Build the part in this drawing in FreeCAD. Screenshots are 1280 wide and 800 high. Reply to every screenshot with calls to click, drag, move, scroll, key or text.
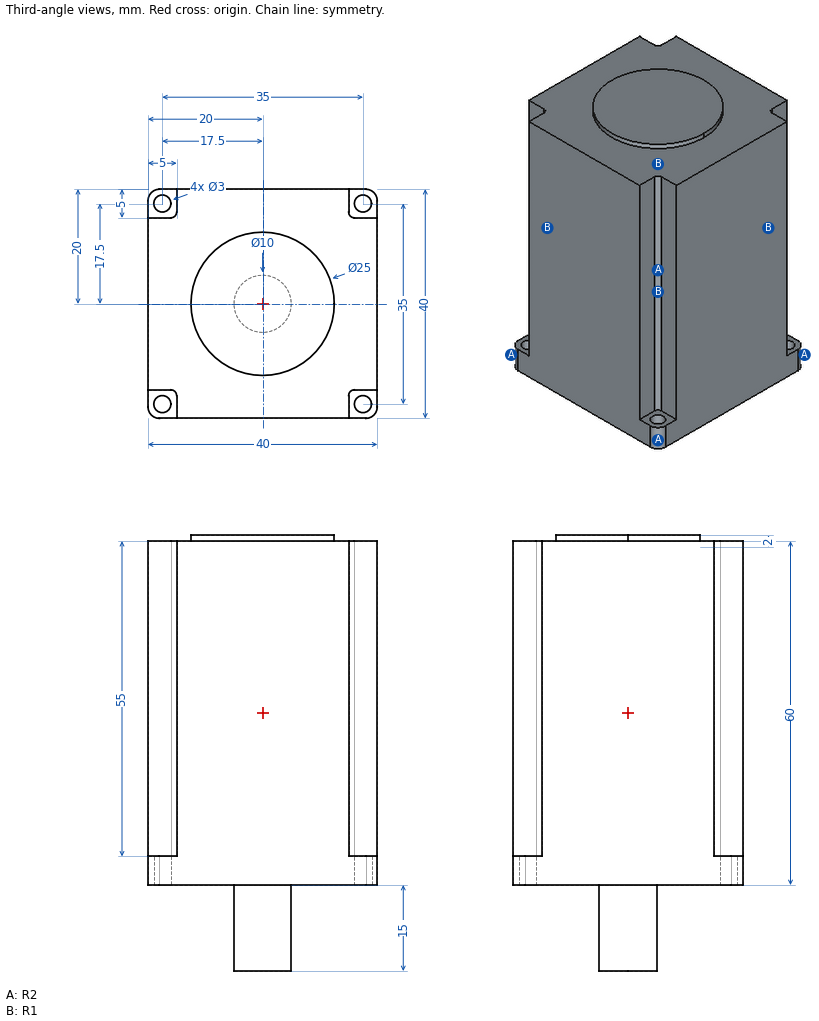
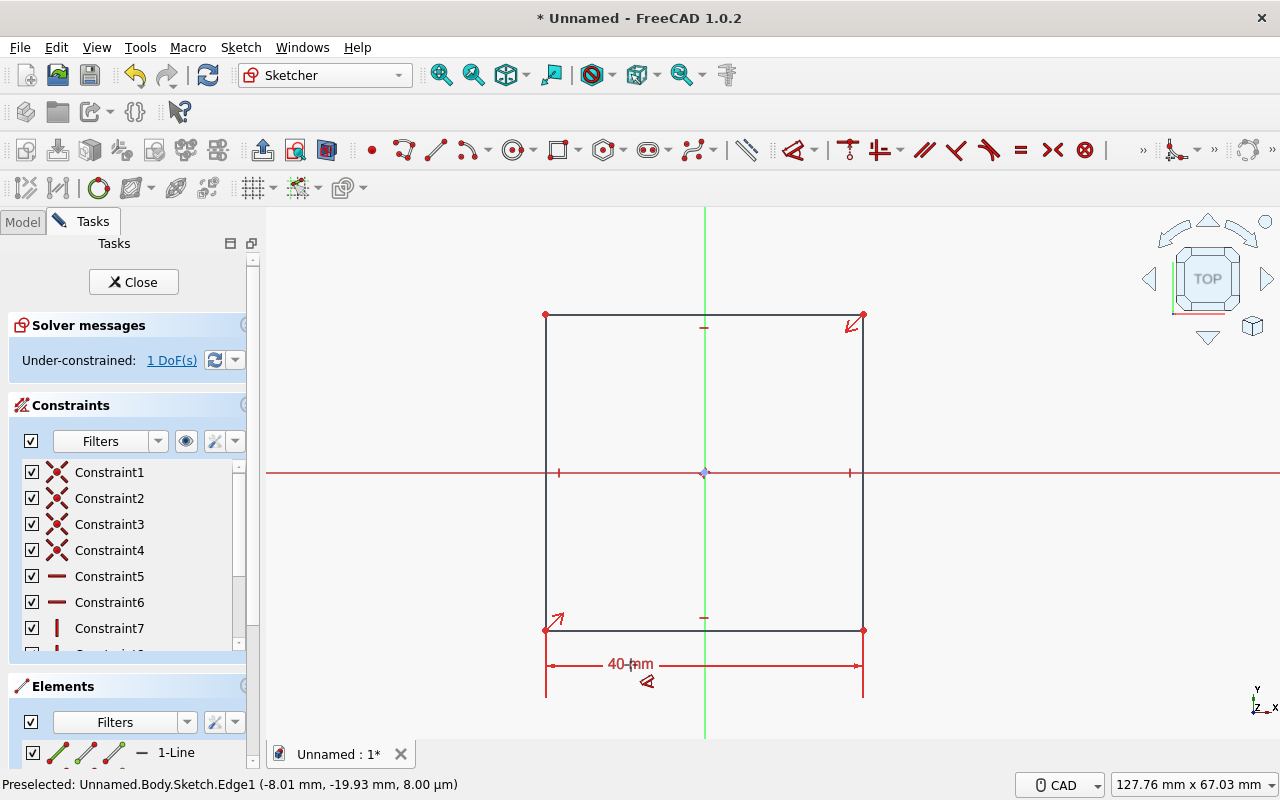
click(863, 536)
click(897, 400)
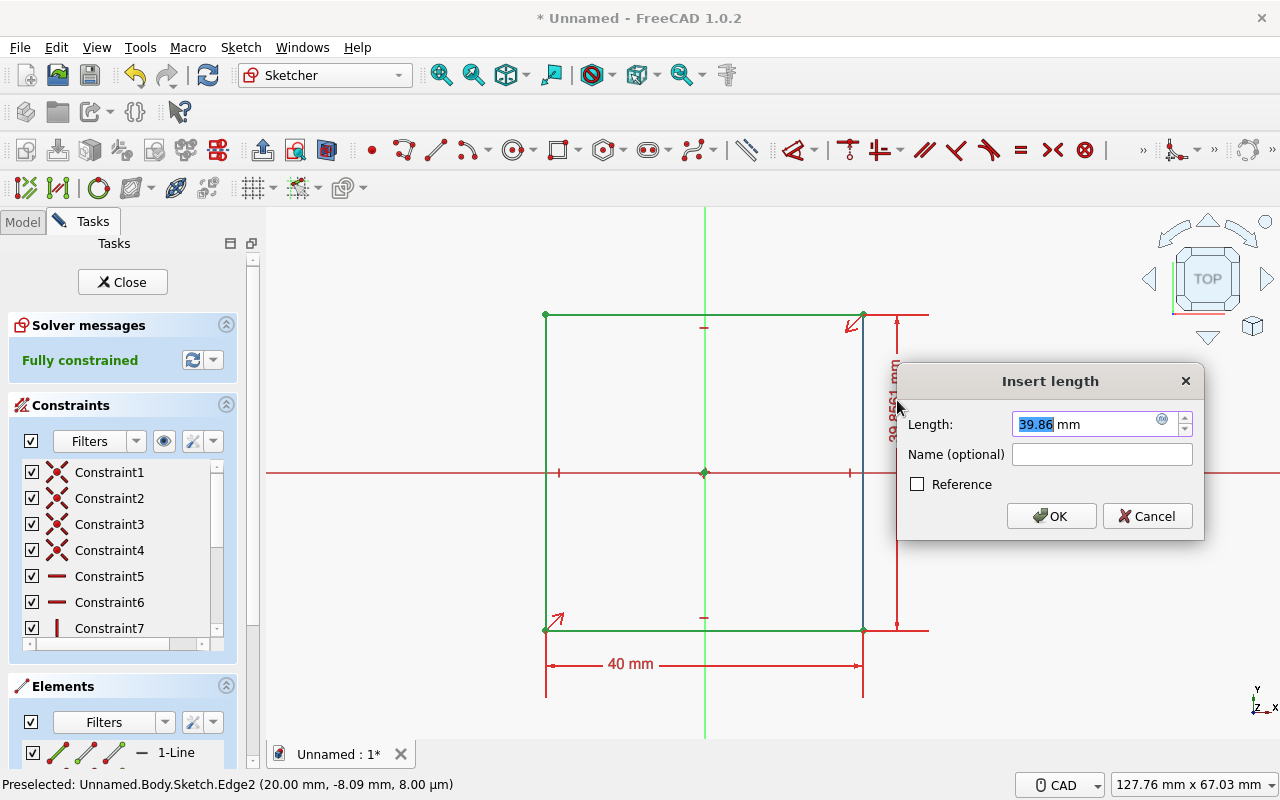
text(40)
key(Return)
key(Escape)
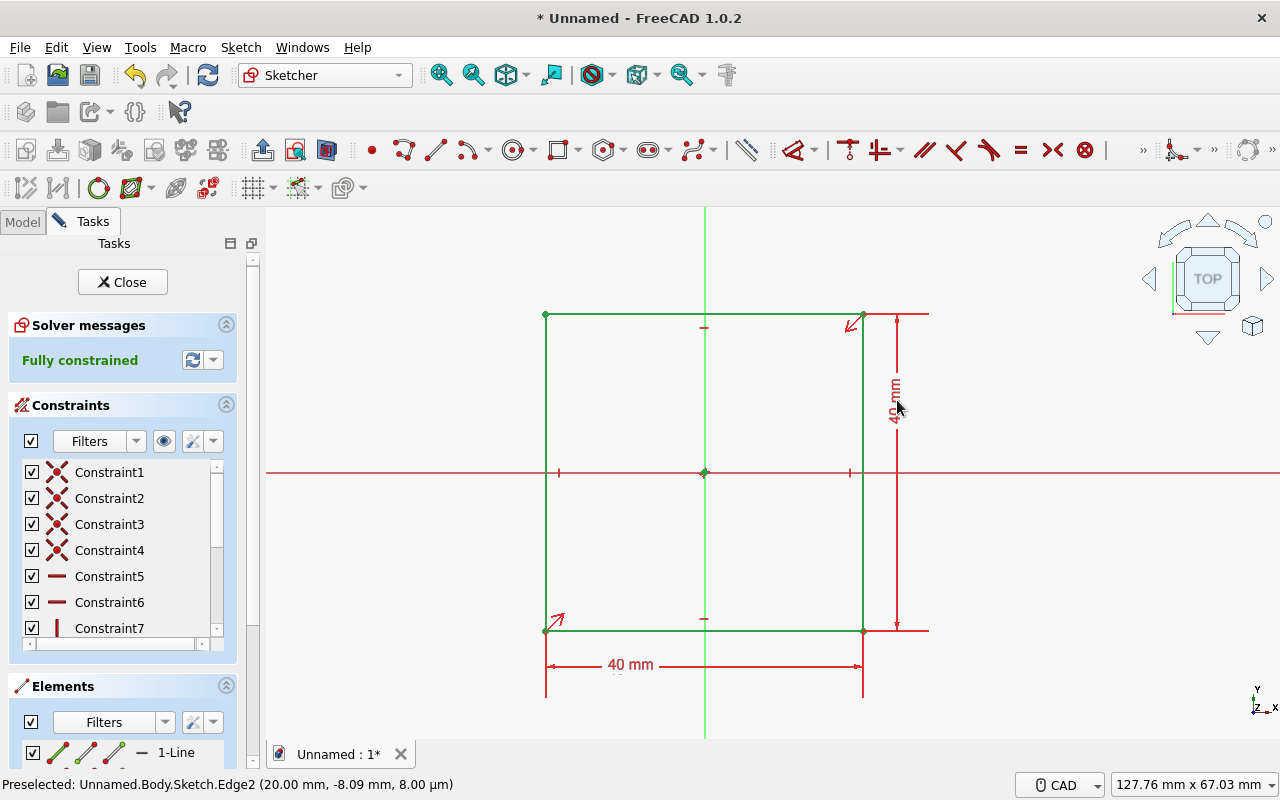
click(123, 282)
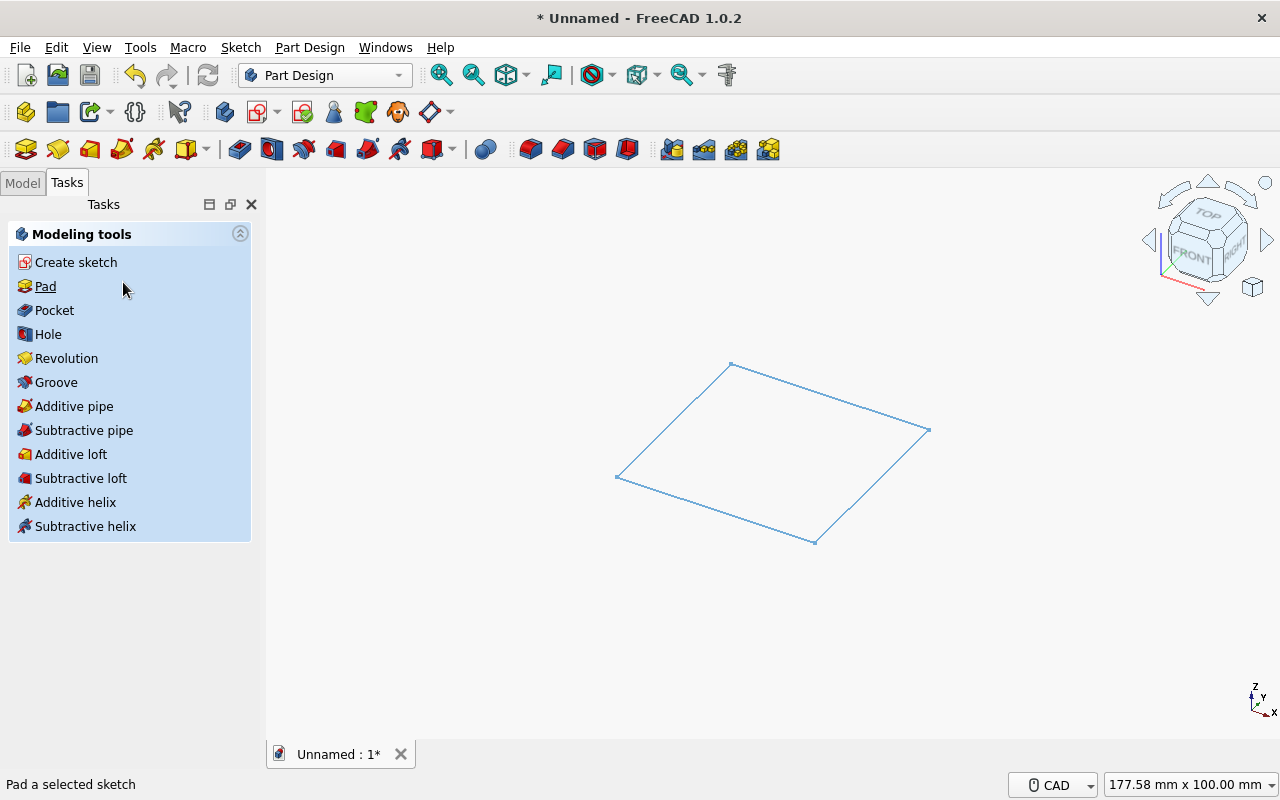
click(26, 150)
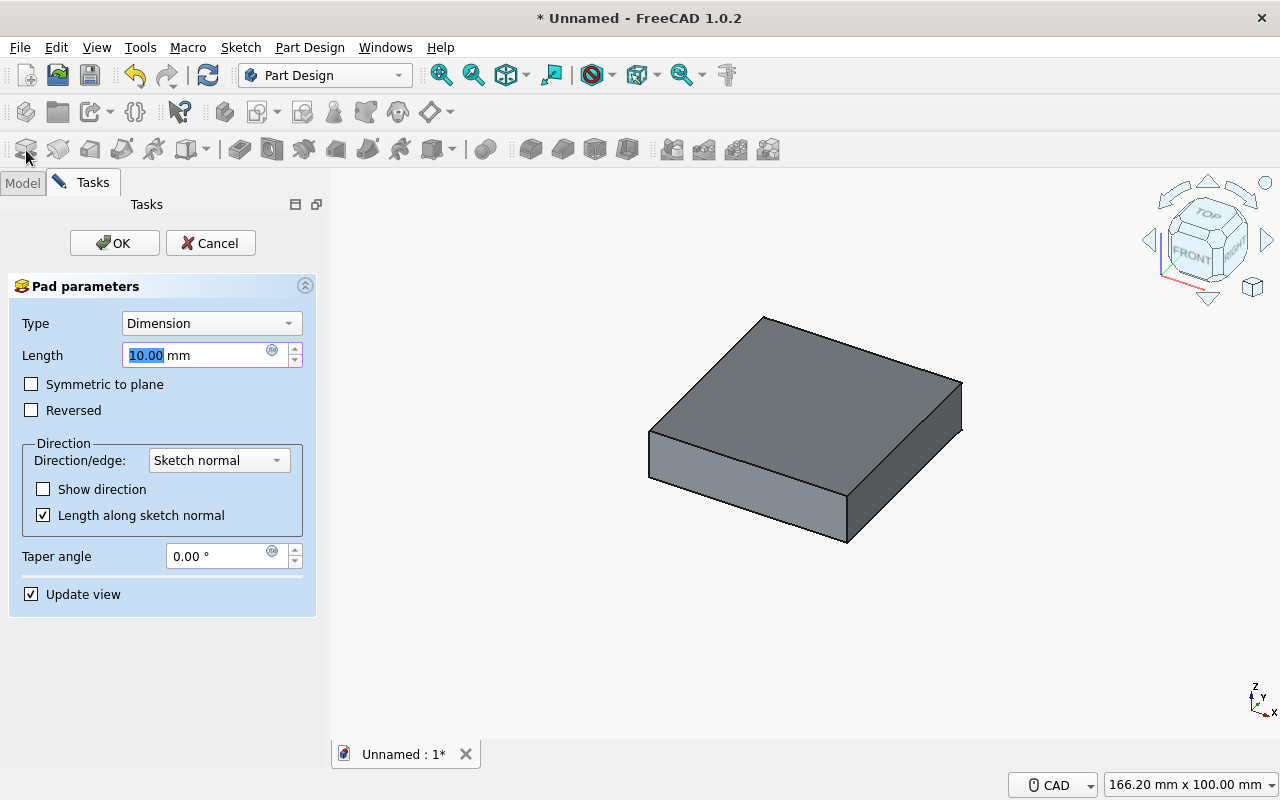
text(60)
key(Tab)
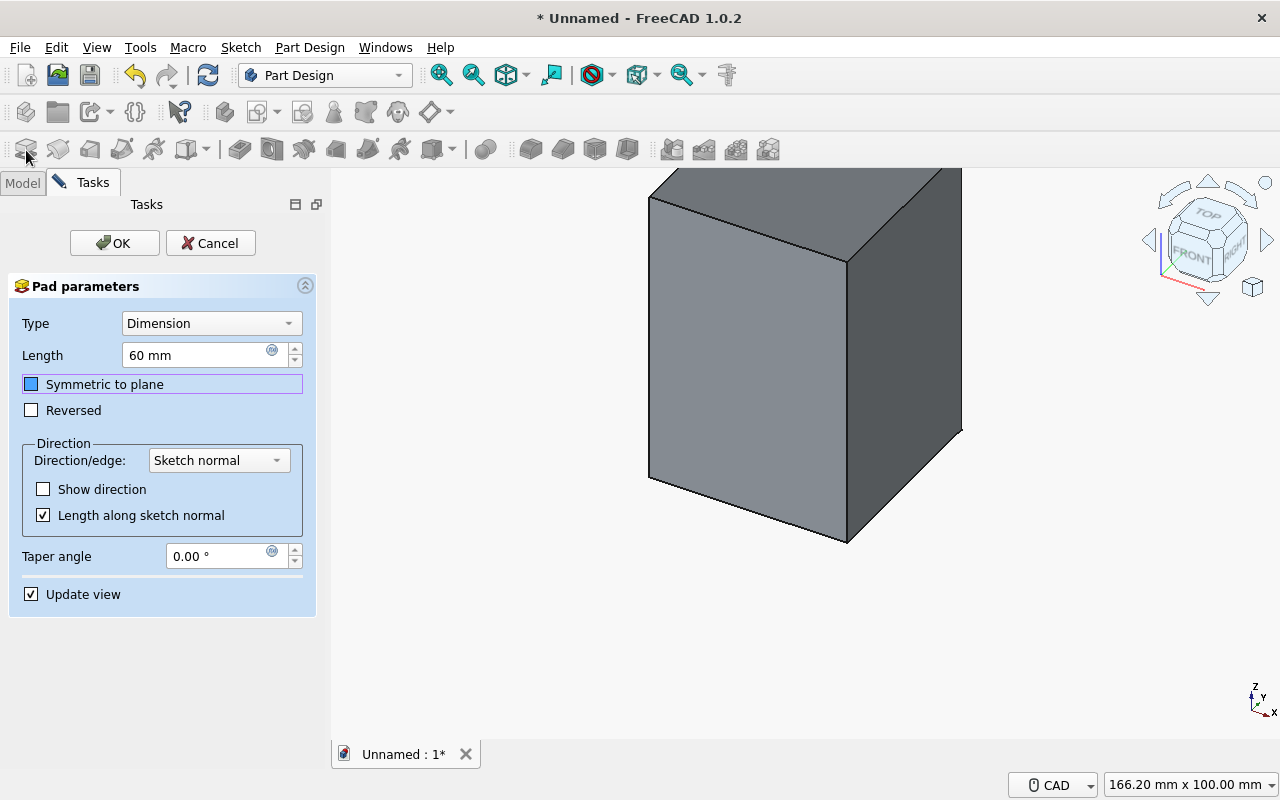
click(30, 384)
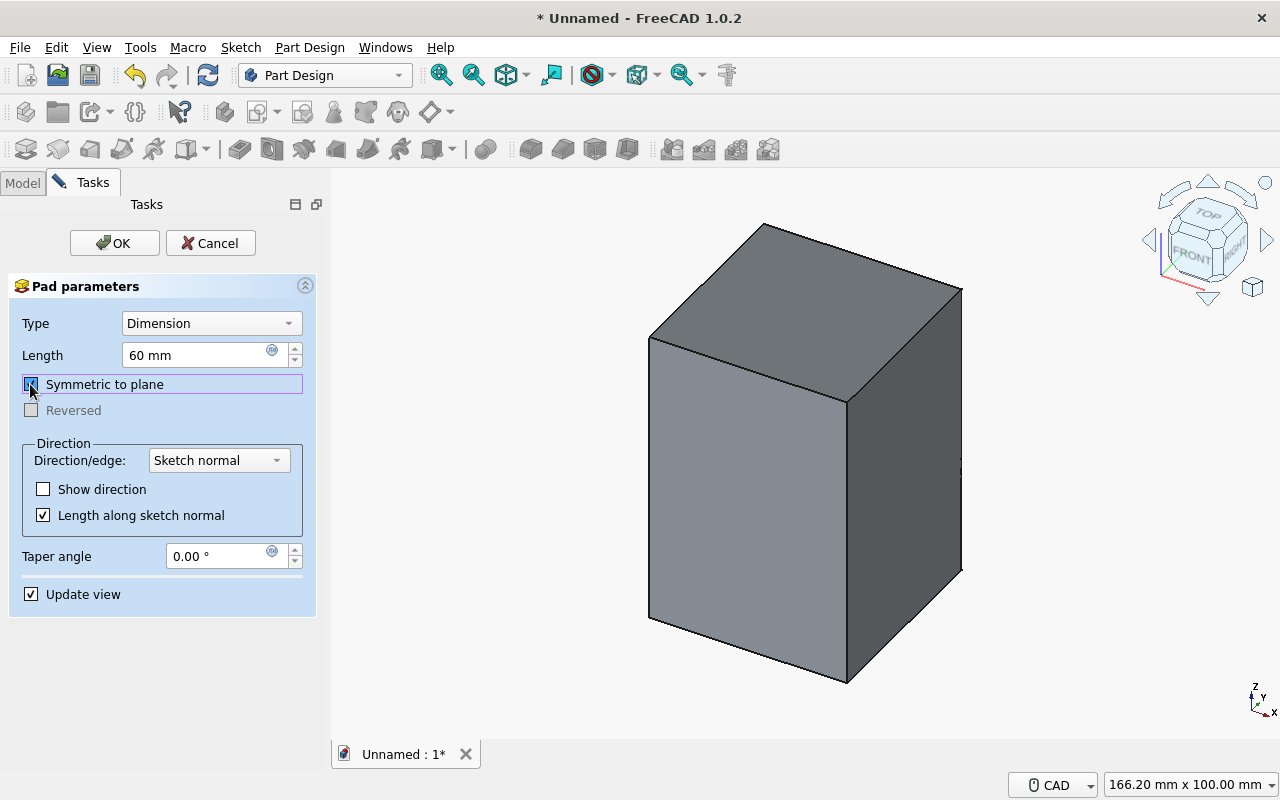
click(115, 243)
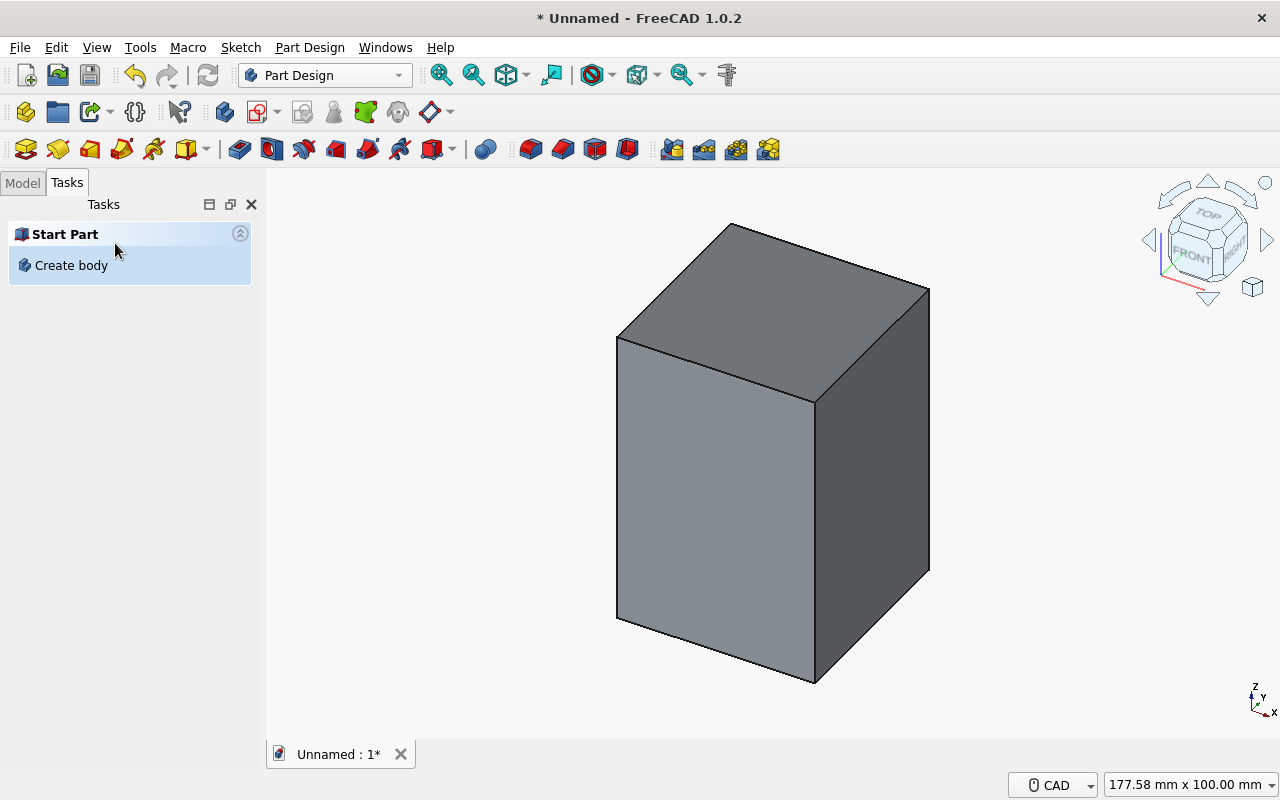
click(773, 312)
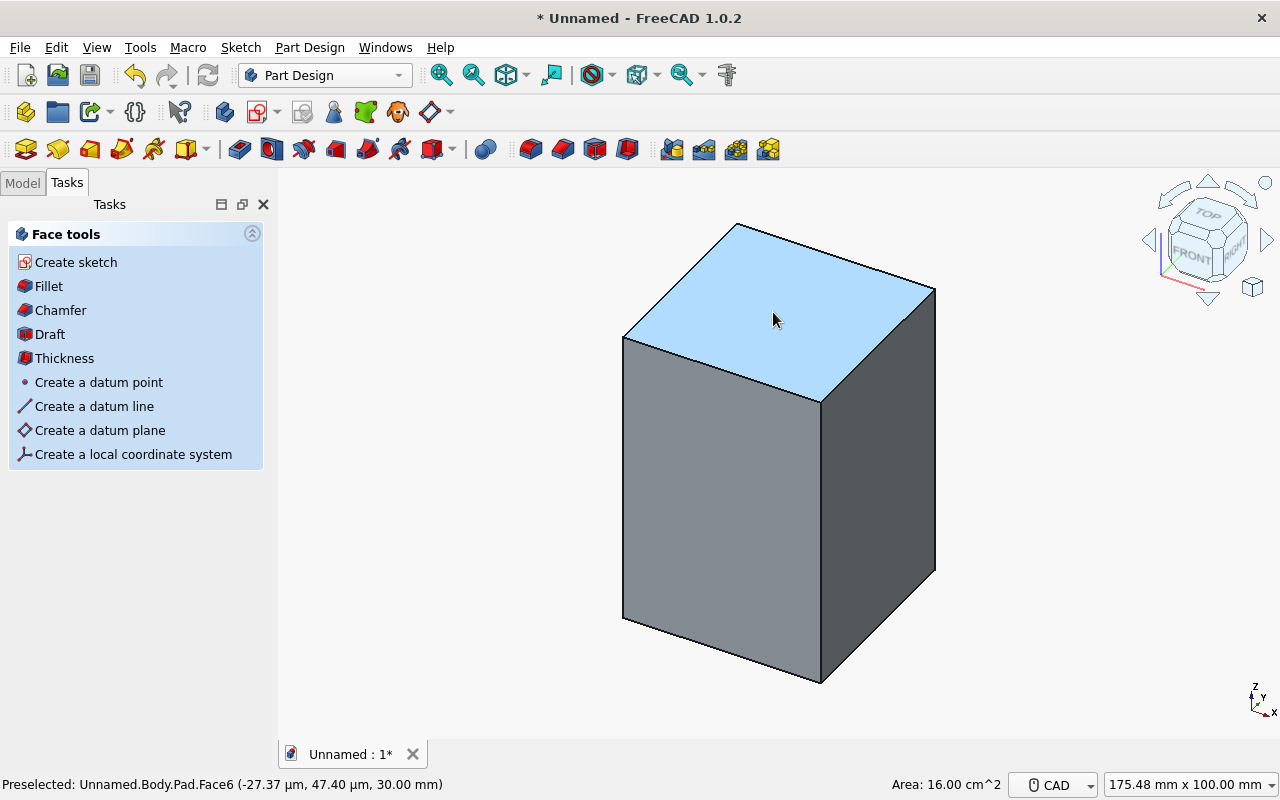
click(258, 112)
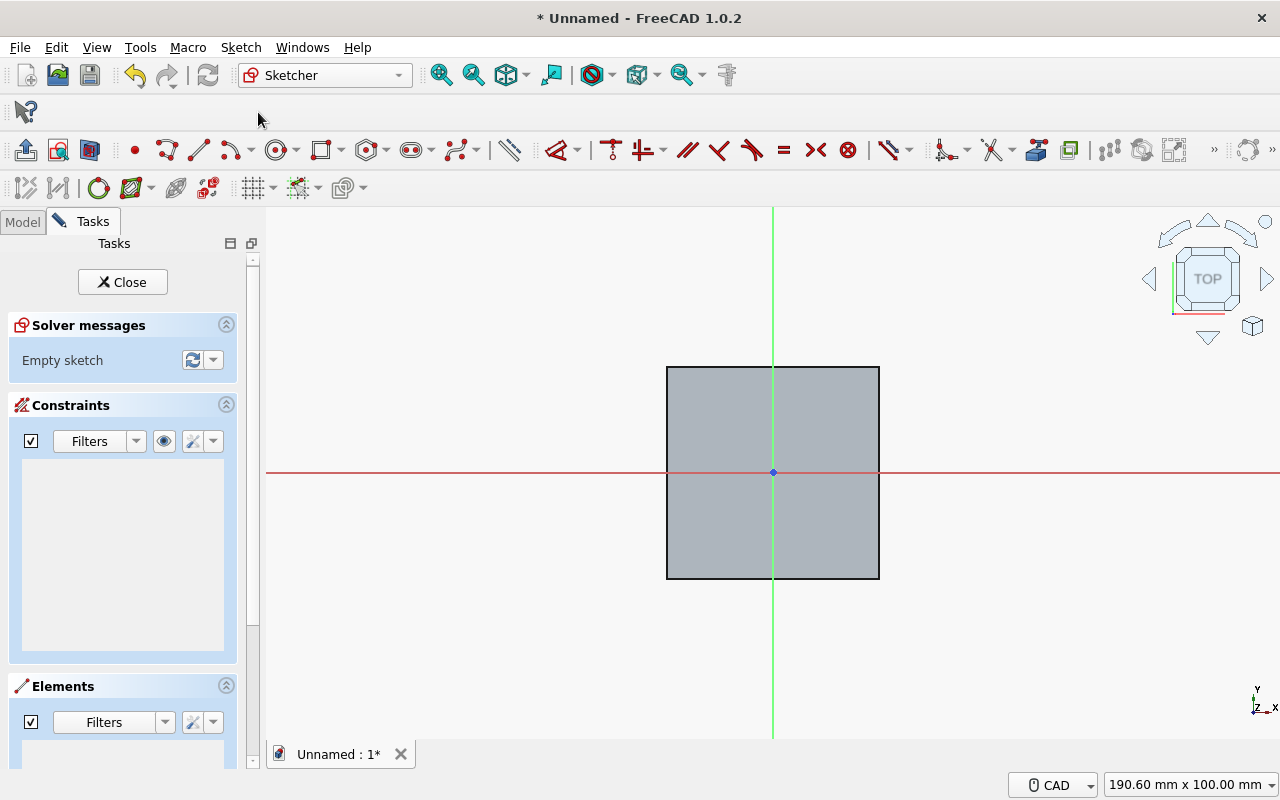
scroll(912, 473, up, 2)